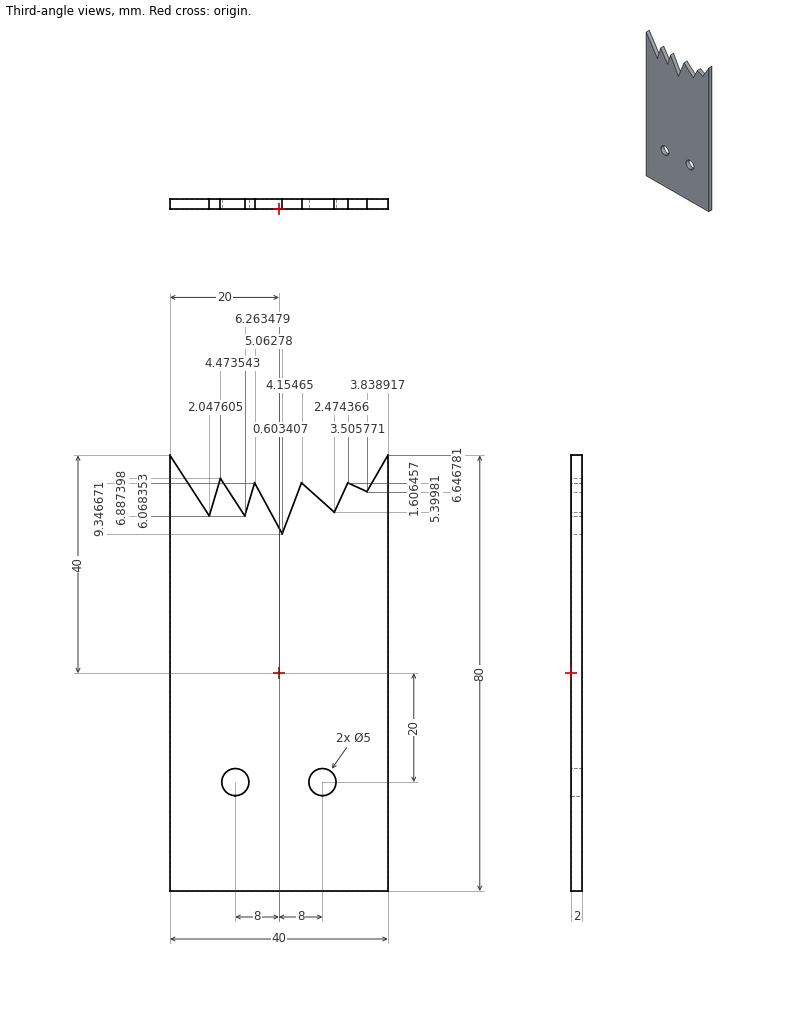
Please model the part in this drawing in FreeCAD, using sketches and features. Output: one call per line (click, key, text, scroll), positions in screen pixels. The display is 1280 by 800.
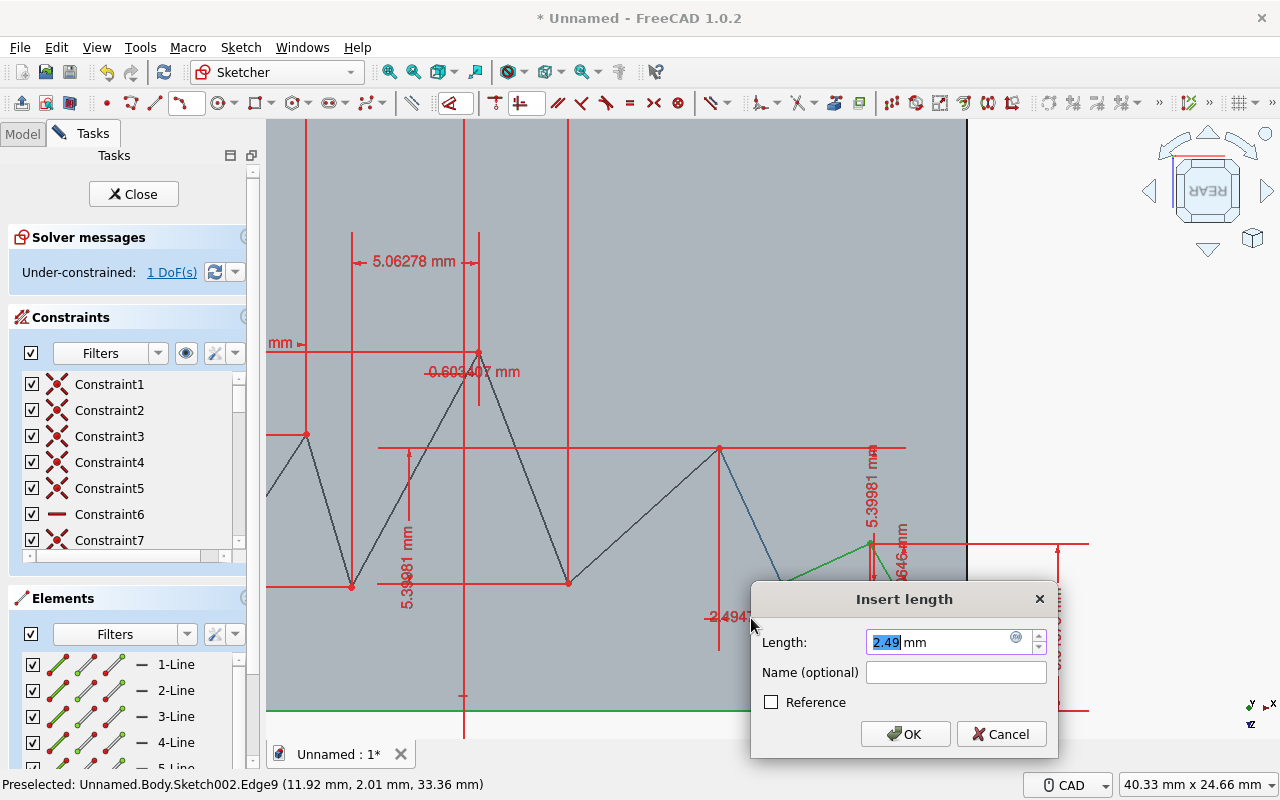
text(2.474366)
key(Return)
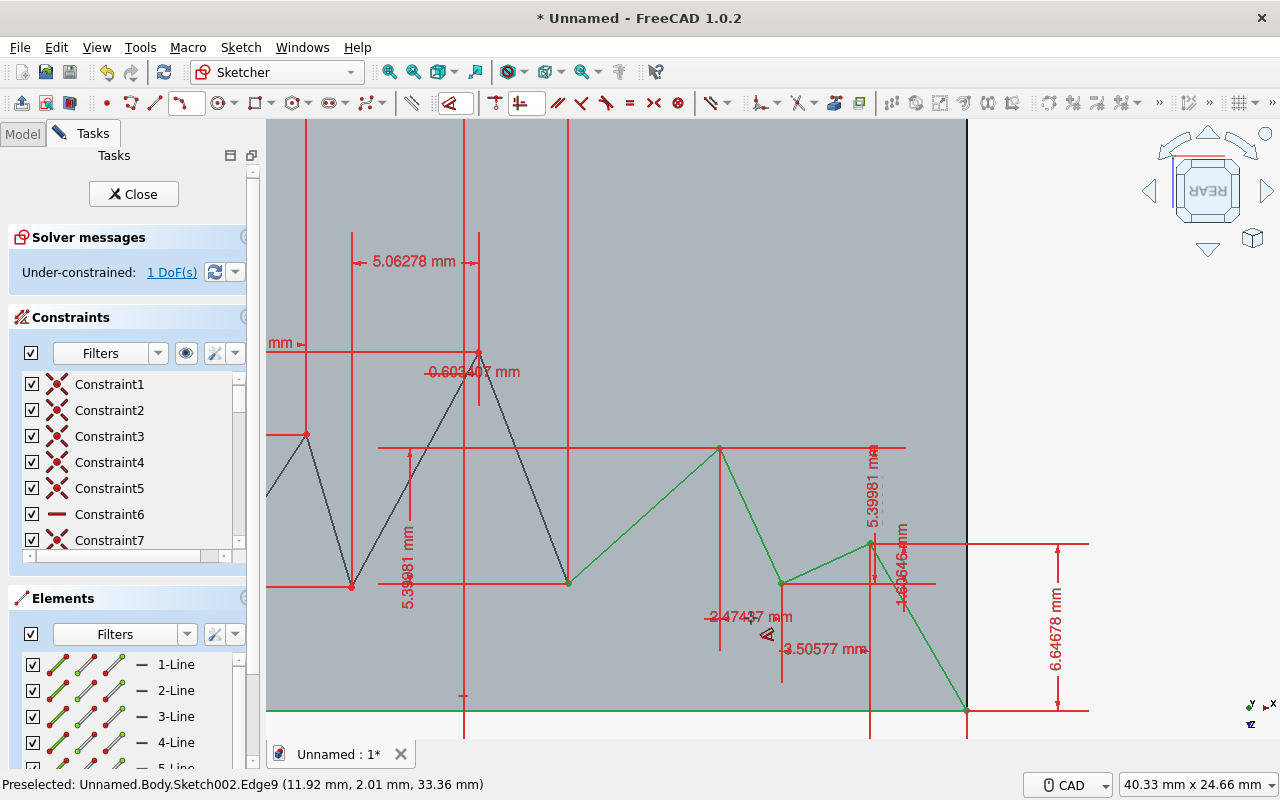
click(541, 514)
click(602, 468)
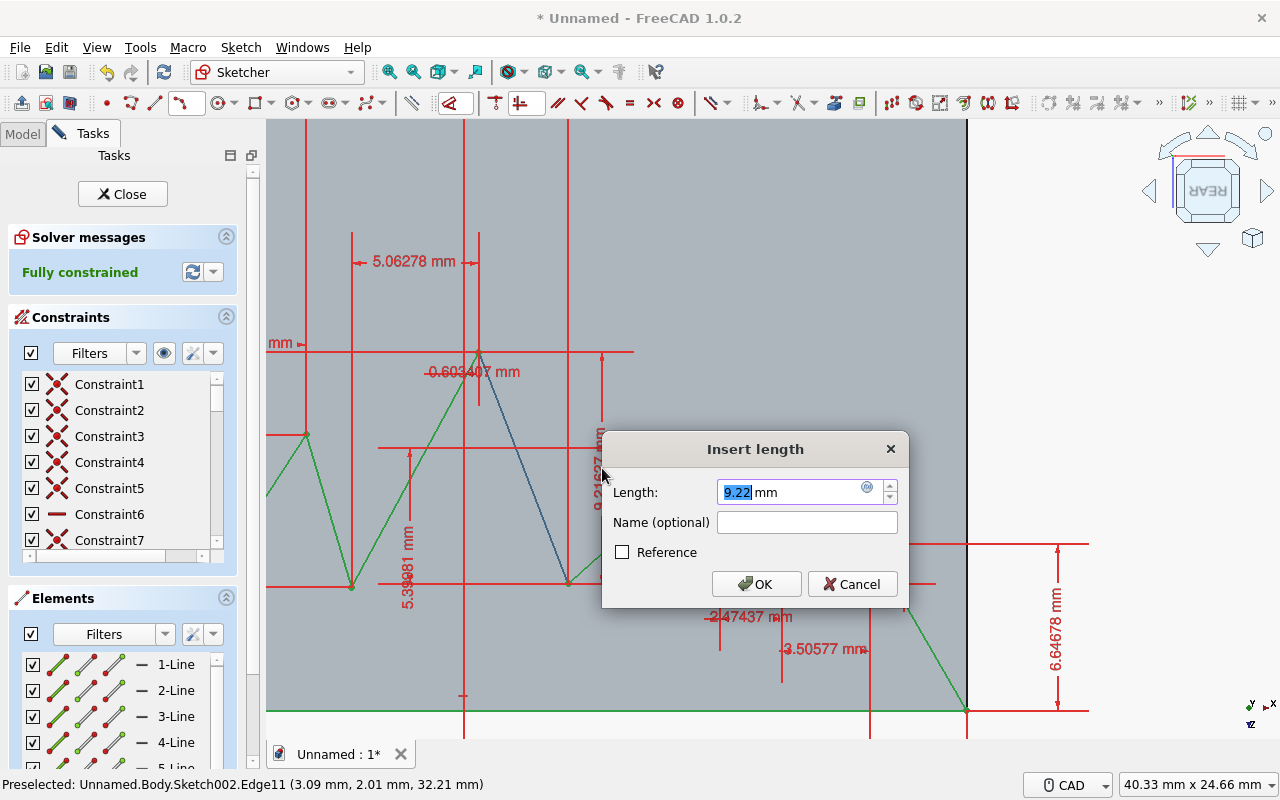
text(9.346671)
key(Return)
key(Escape)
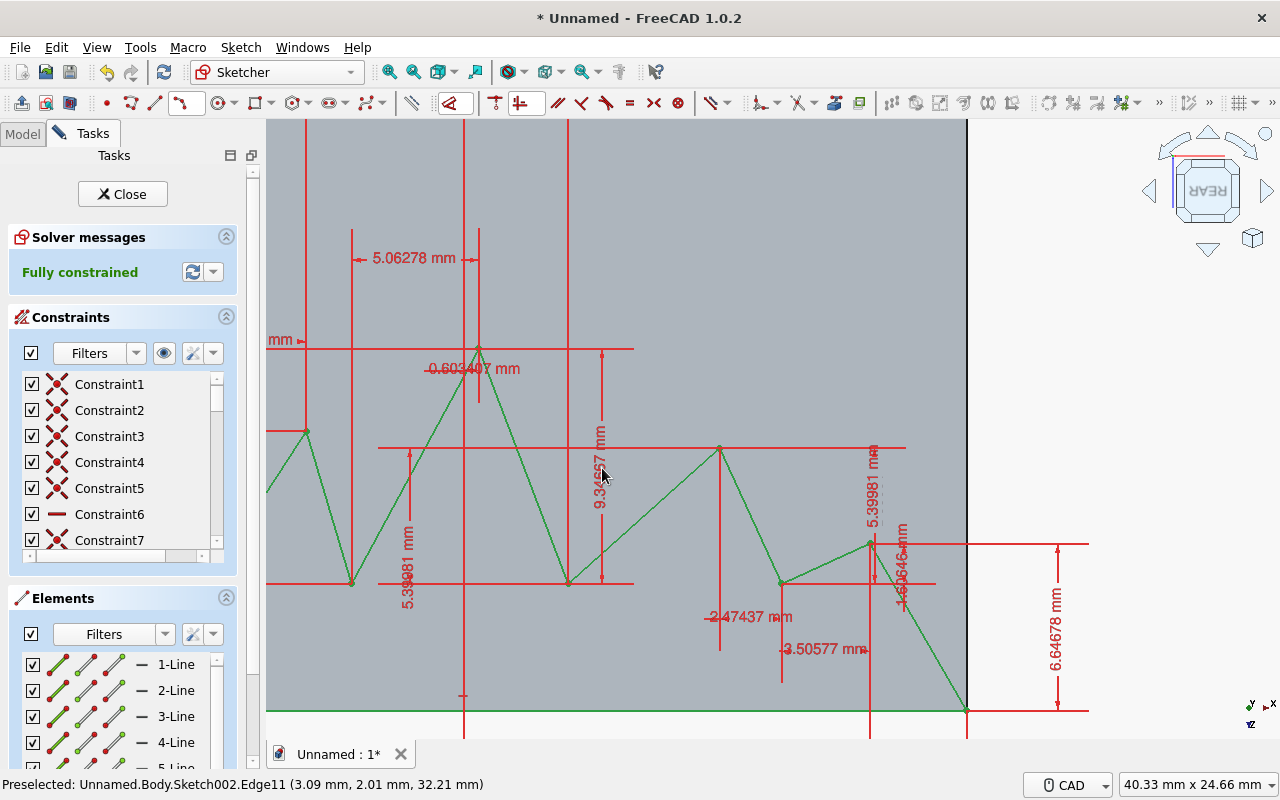
click(123, 194)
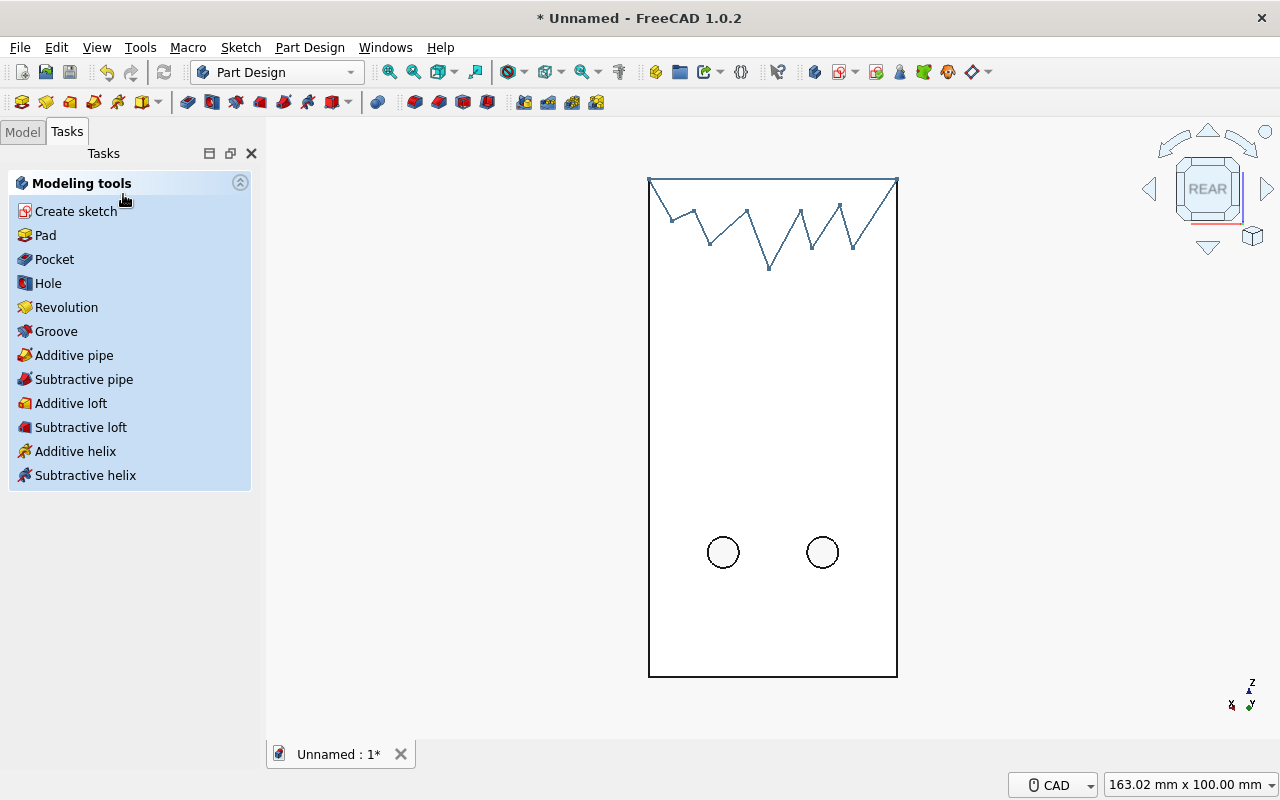
click(188, 102)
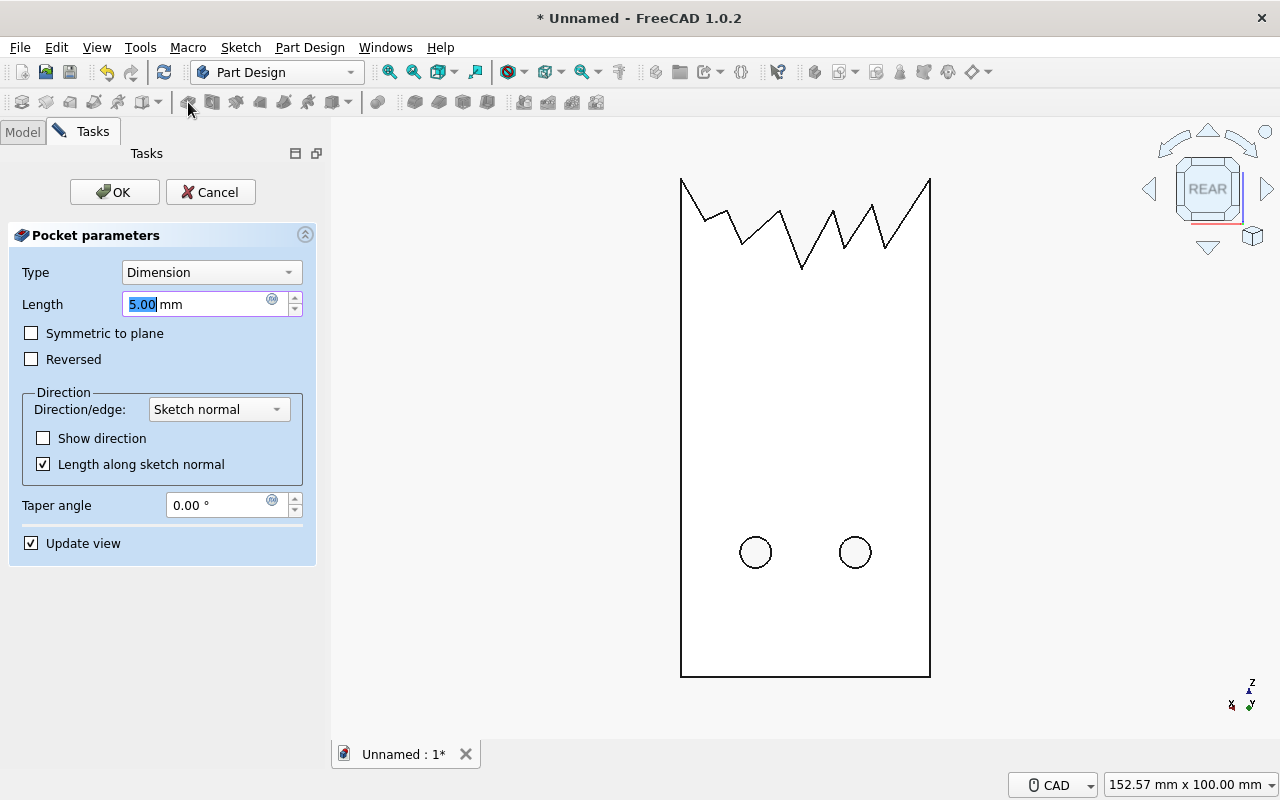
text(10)
key(Tab)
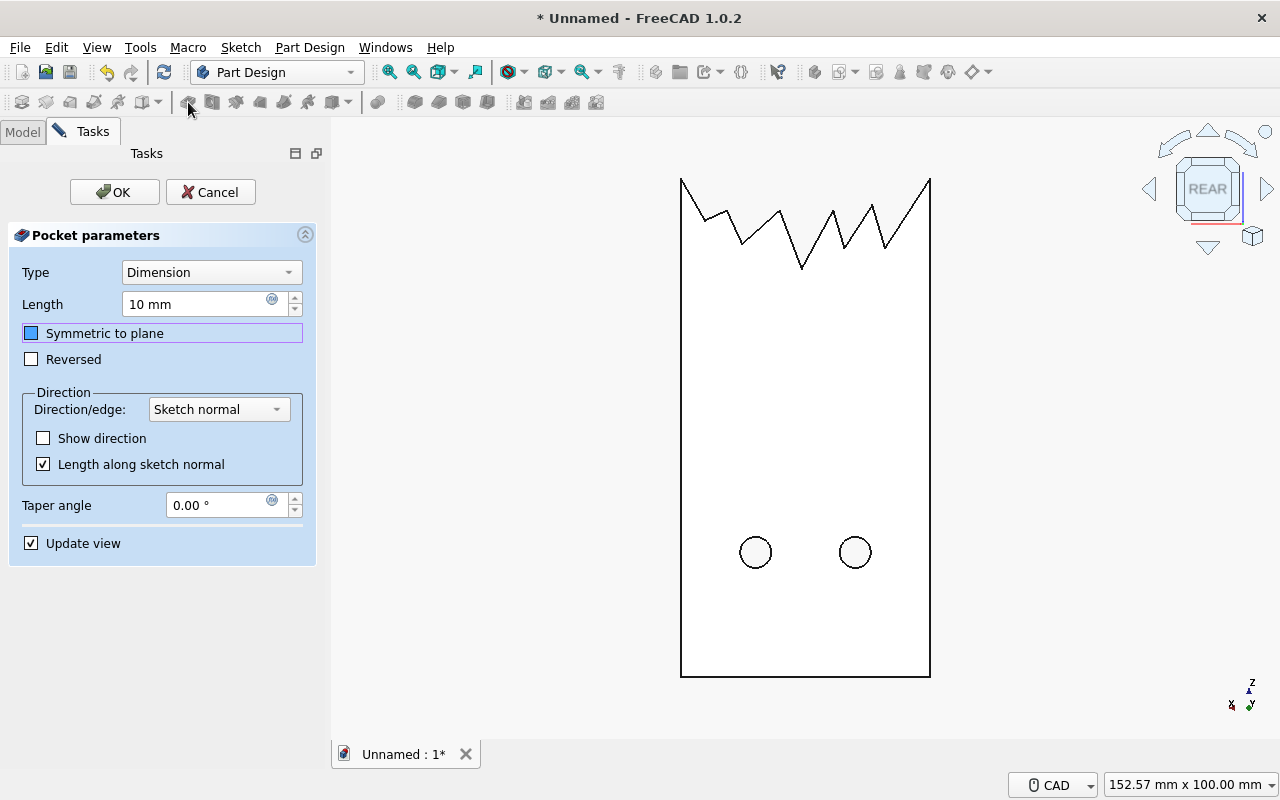
click(115, 192)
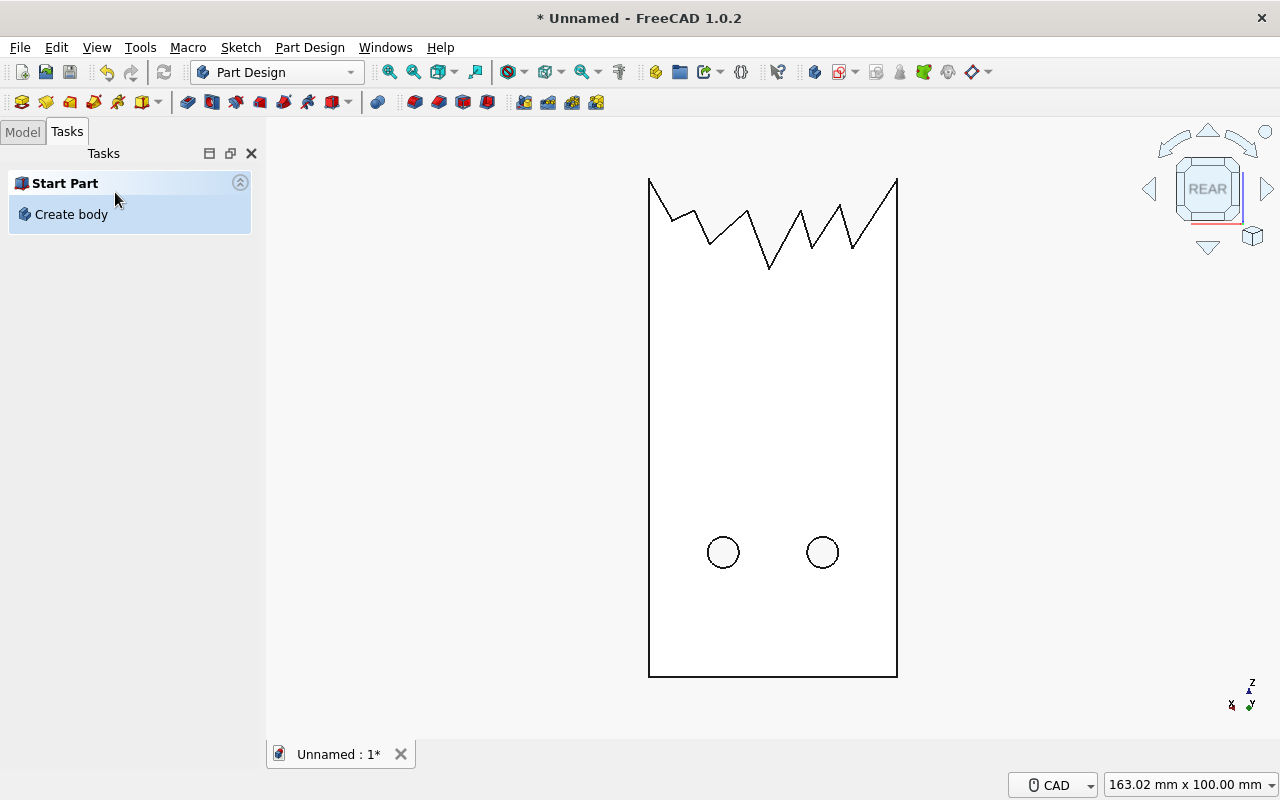
key(0)